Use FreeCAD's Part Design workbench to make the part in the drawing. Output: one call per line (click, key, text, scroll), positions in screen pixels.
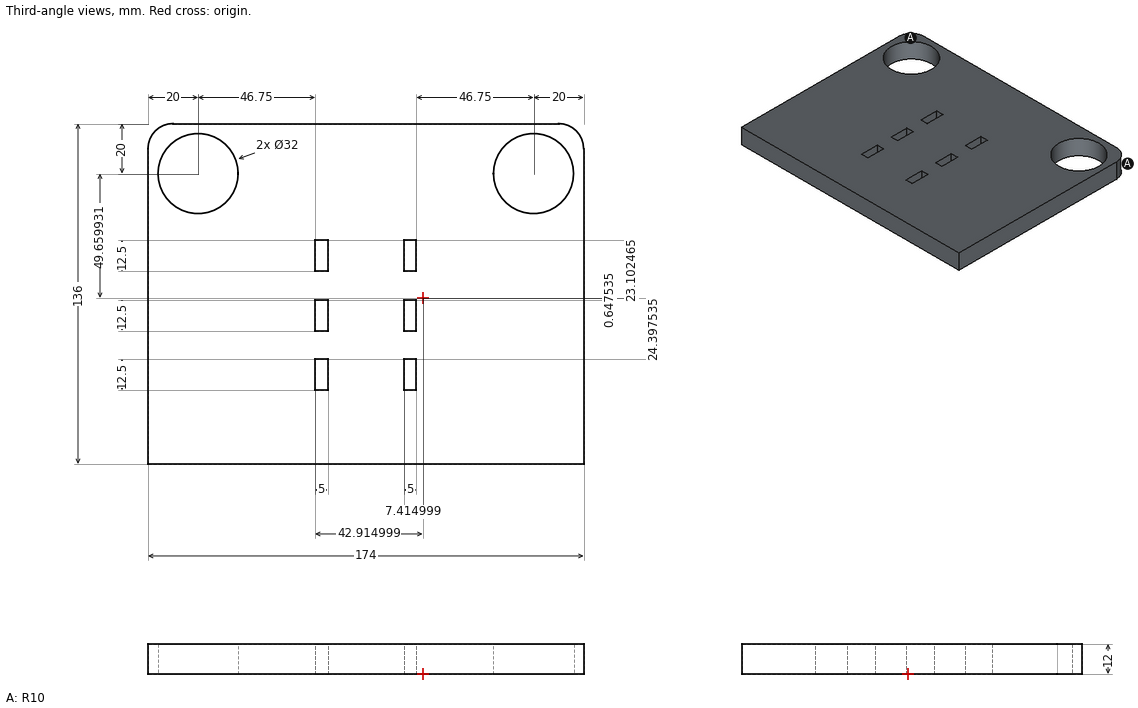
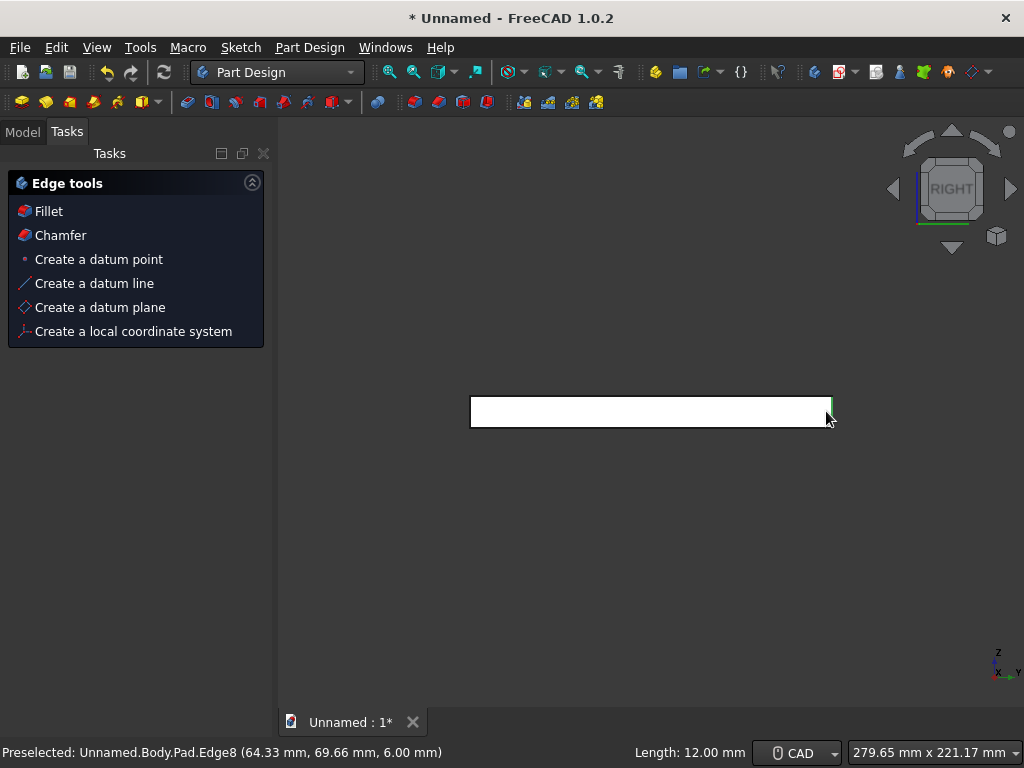
key(5)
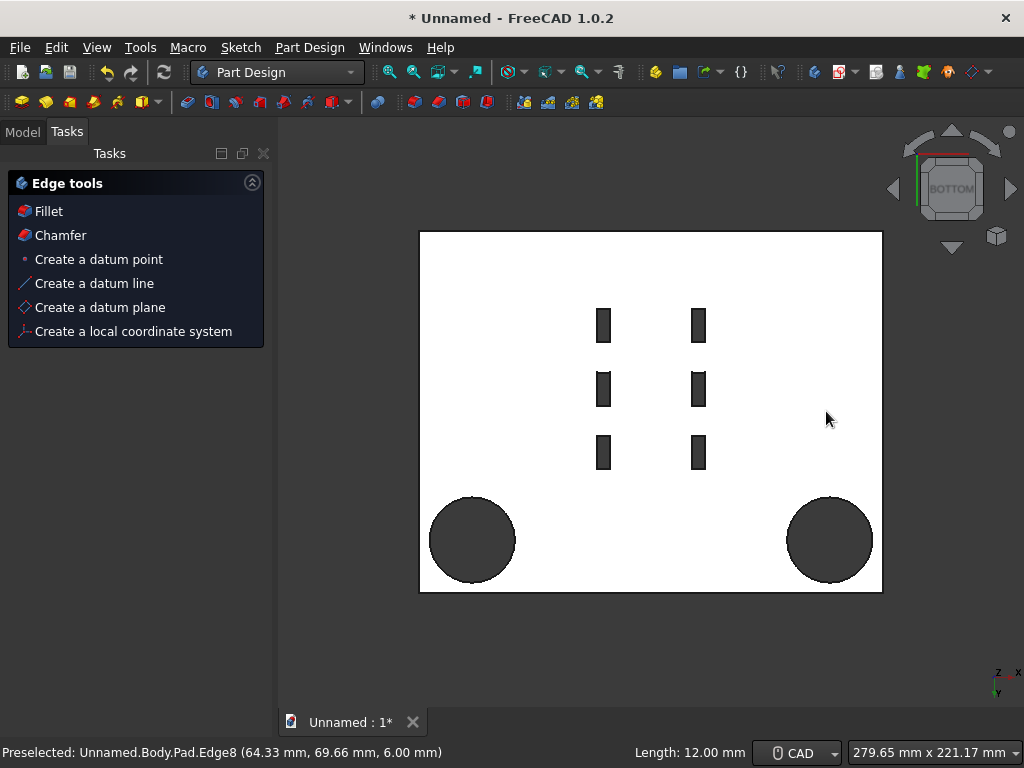
key(4)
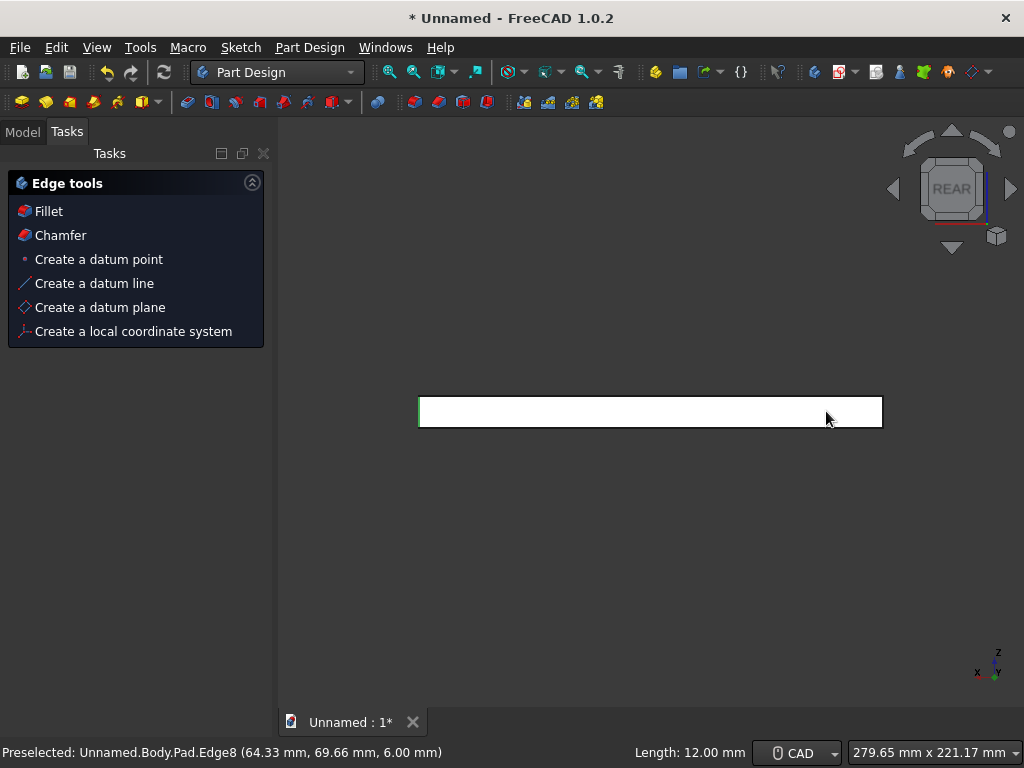
click(883, 411, ctrl)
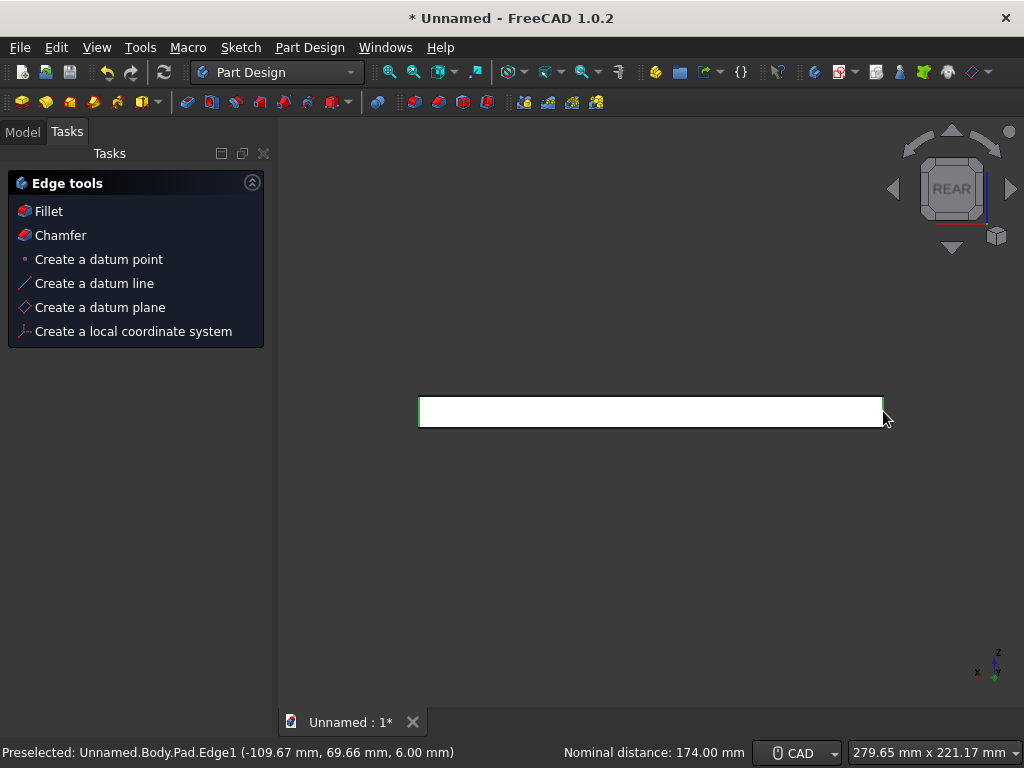
click(416, 102)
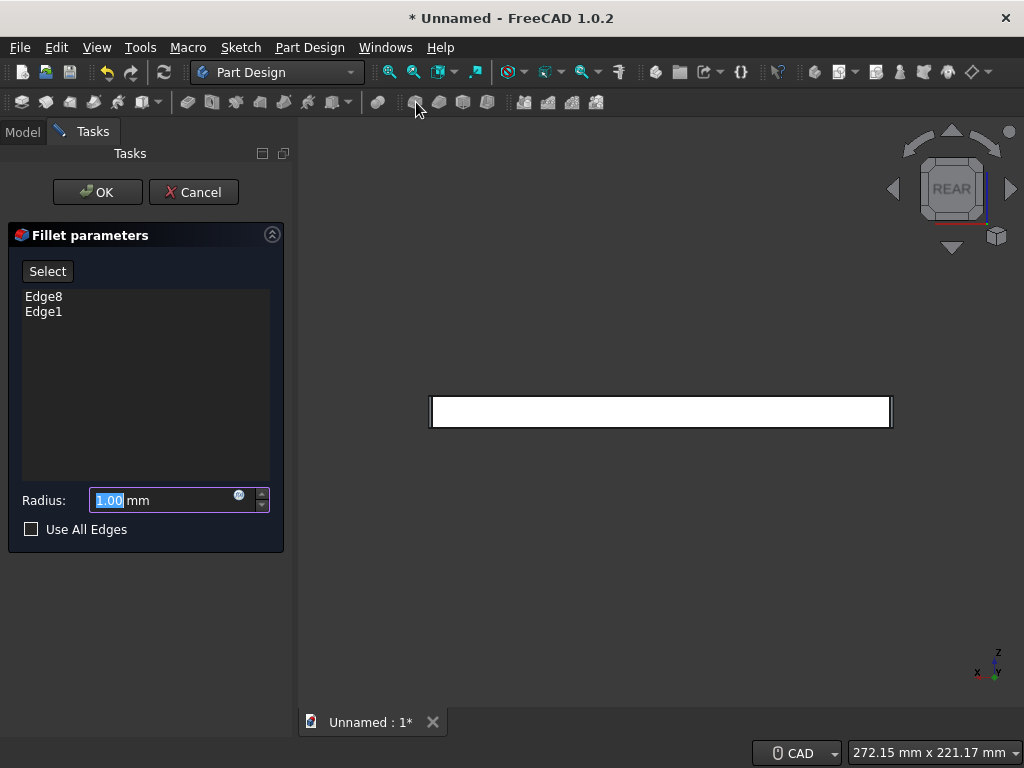
text(10)
key(Tab)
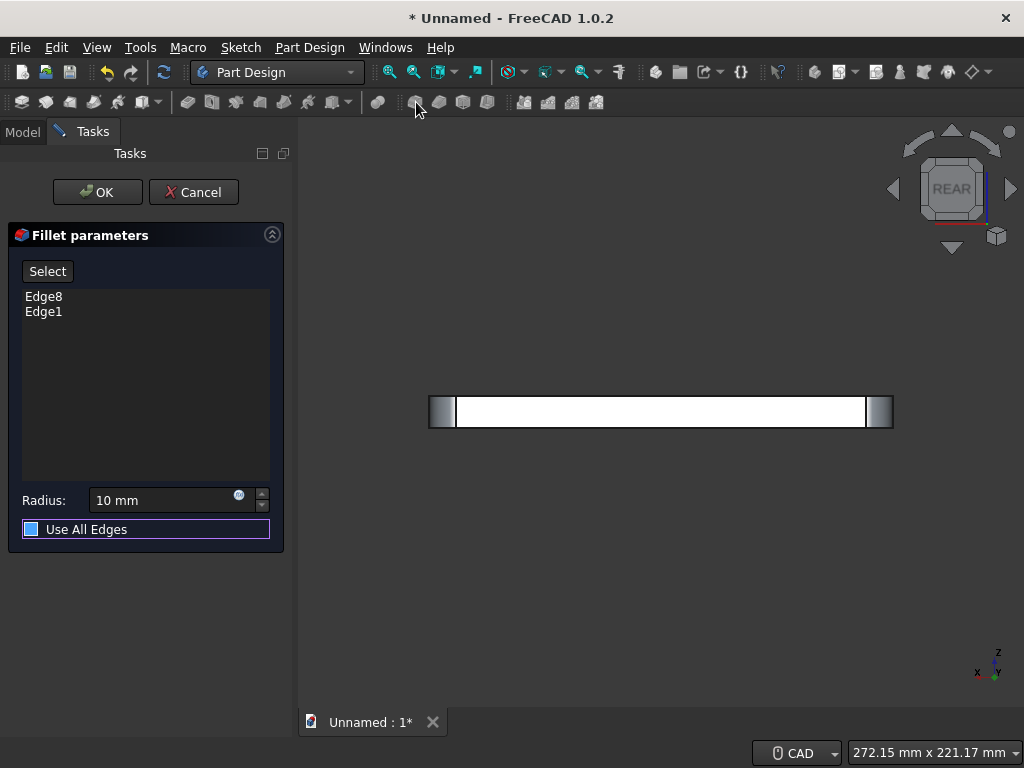
click(98, 192)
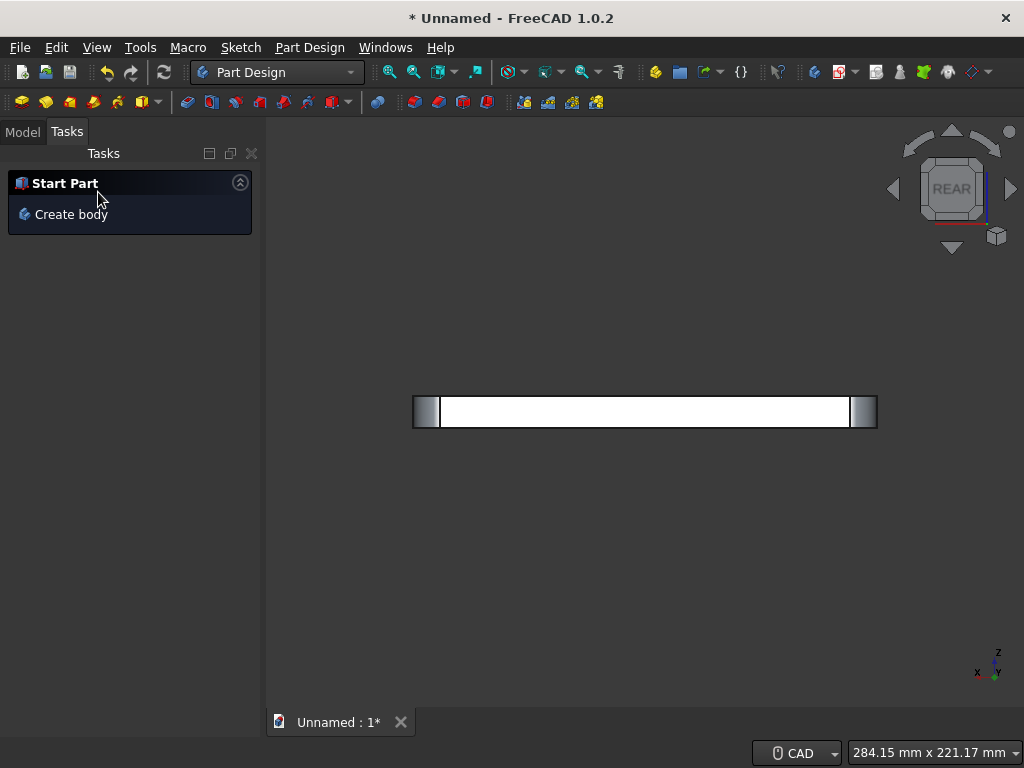
key(0)